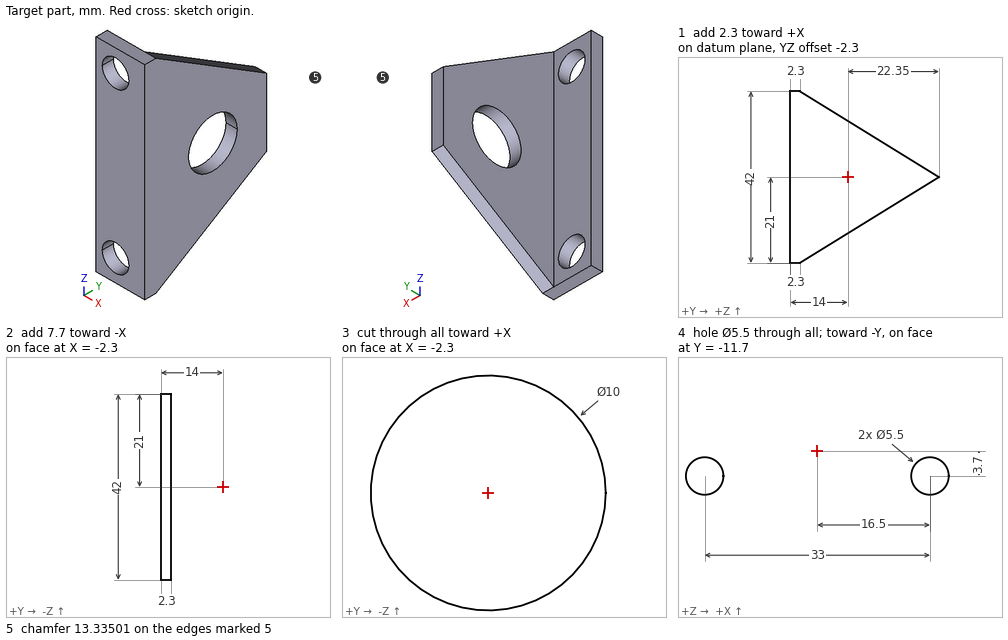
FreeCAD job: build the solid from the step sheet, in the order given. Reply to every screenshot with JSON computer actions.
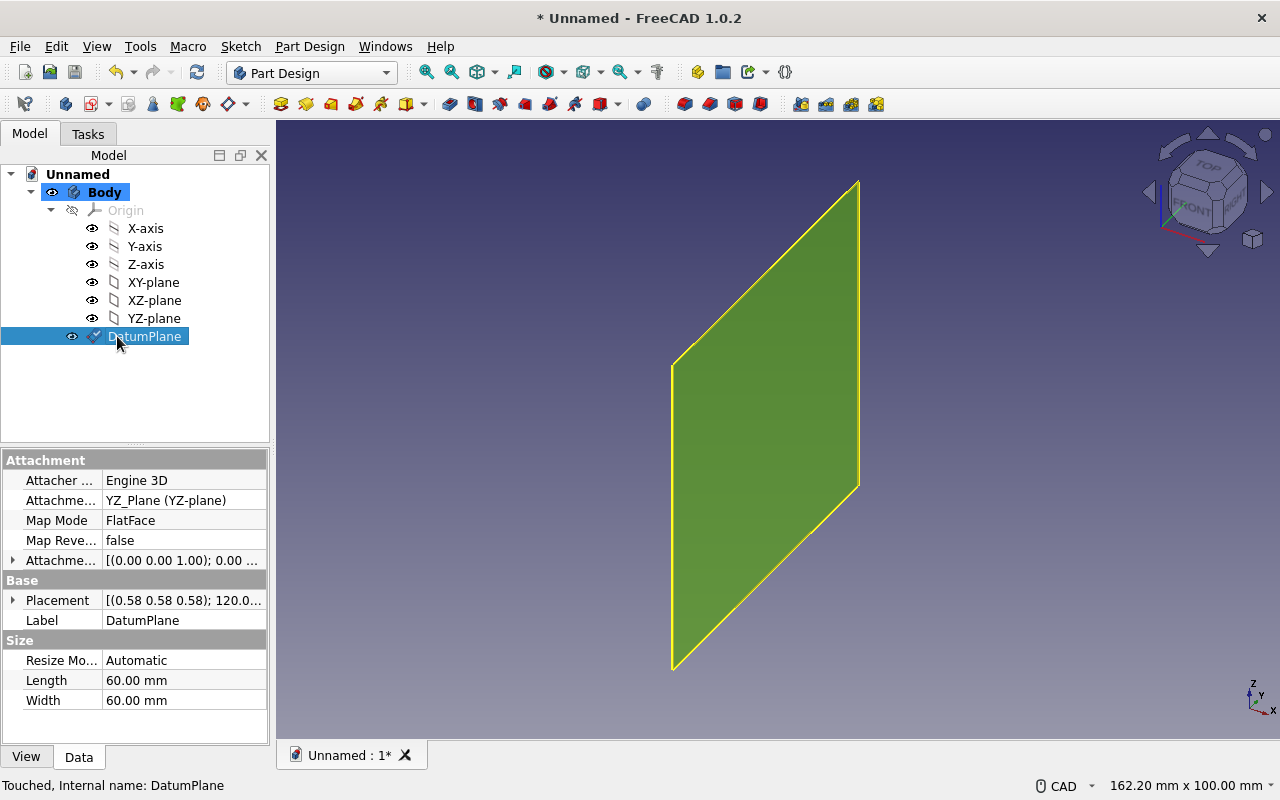
{"action": "left_click", "coordinate": [90, 104]}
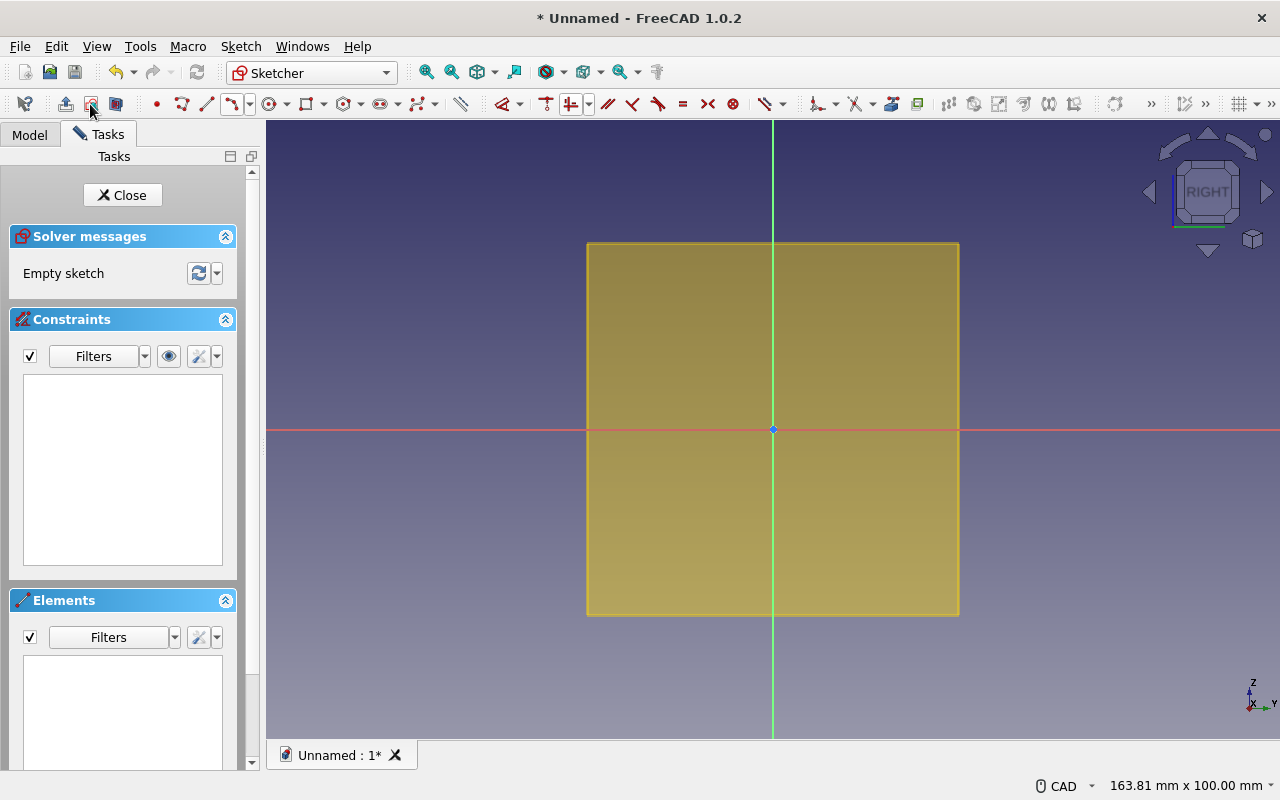
{"action": "scroll", "coordinate": [991, 429], "scroll_direction": "up", "scroll_amount": 2}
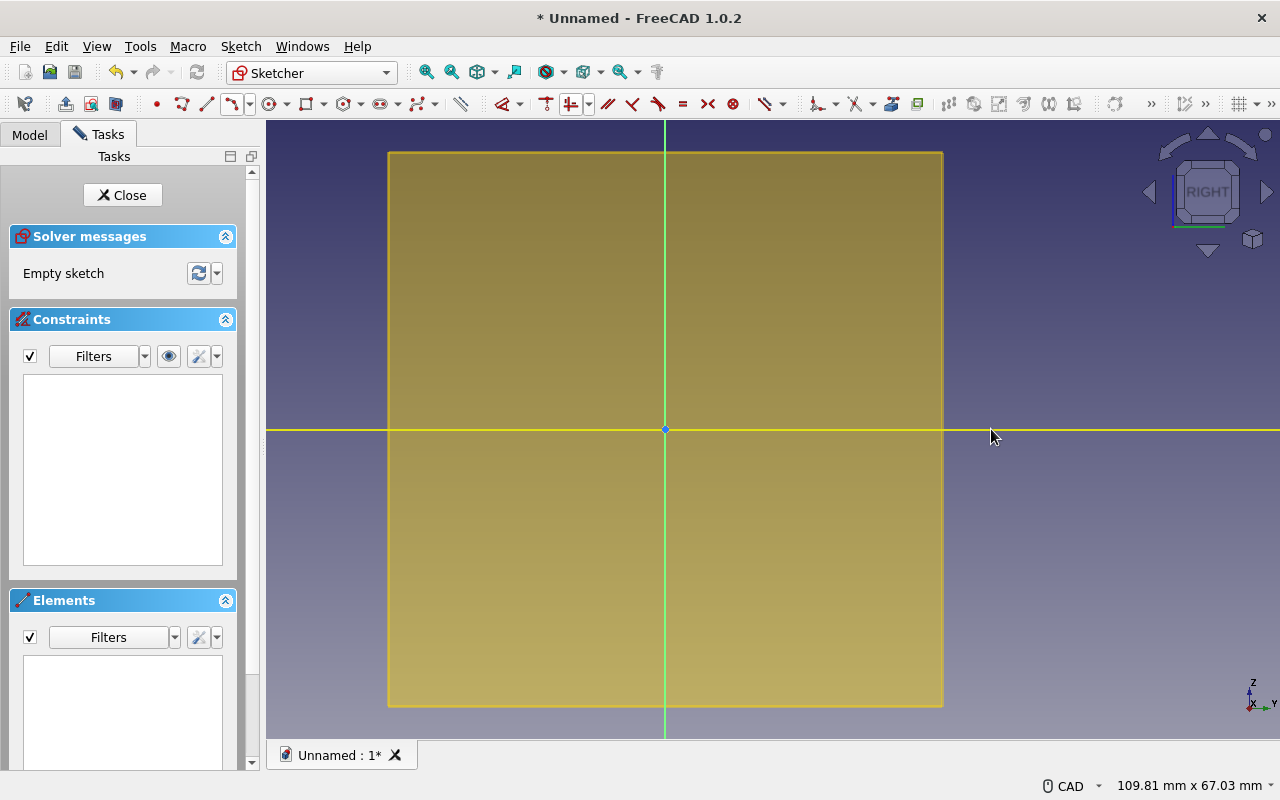
{"action": "key", "text": "g m"}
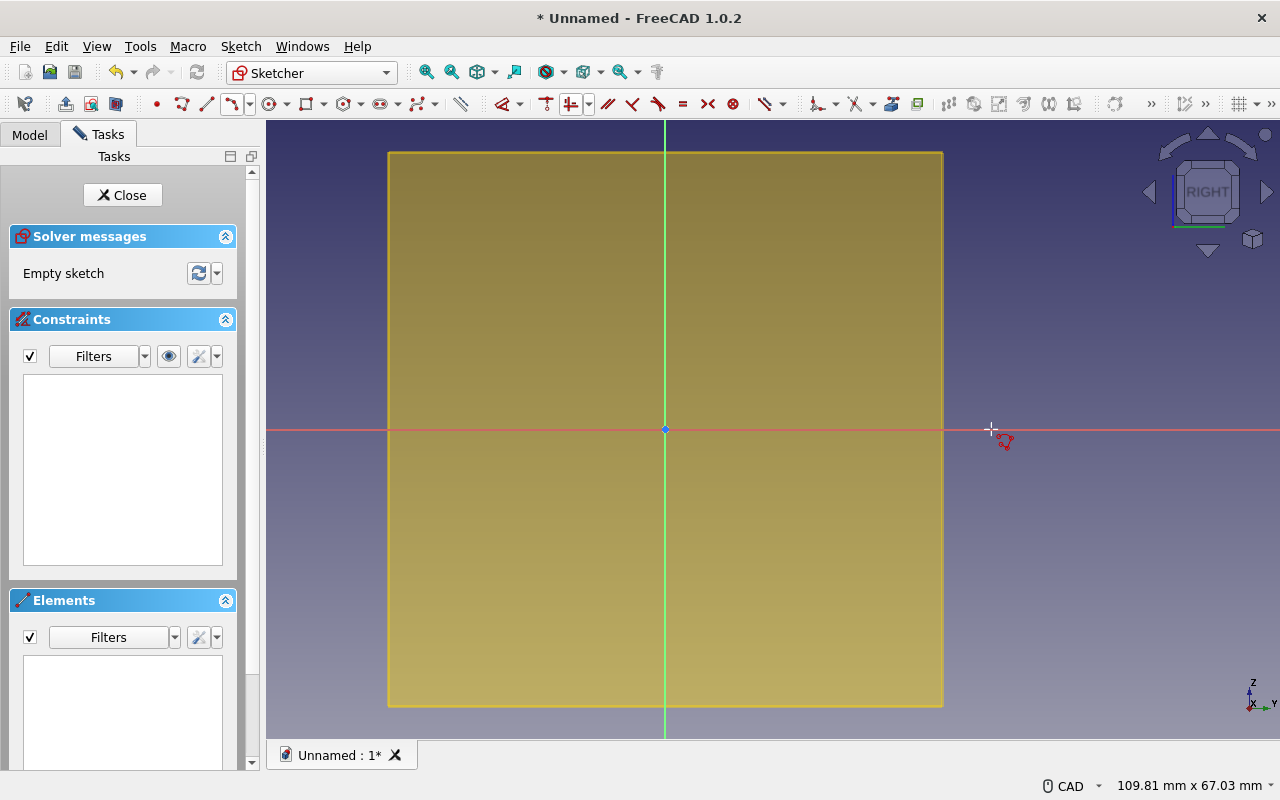
{"action": "left_click", "coordinate": [872, 430]}
{"action": "left_click", "coordinate": [557, 623]}
{"action": "left_click", "coordinate": [536, 623]}
{"action": "left_click", "coordinate": [536, 236]}
{"action": "left_click", "coordinate": [557, 236]}
{"action": "left_click", "coordinate": [872, 430]}
{"action": "key", "text": "Escape"}
{"action": "key", "text": "Escape"}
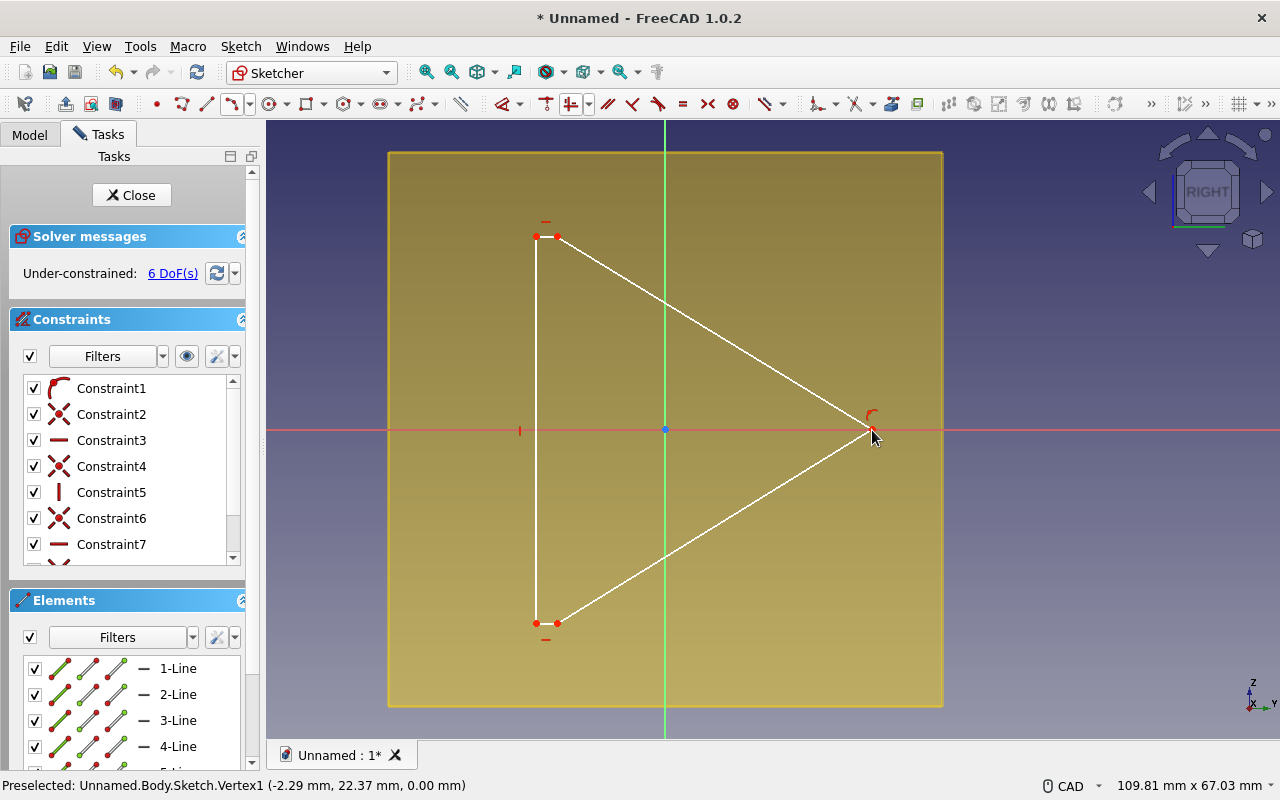
{"action": "left_click", "coordinate": [536, 508]}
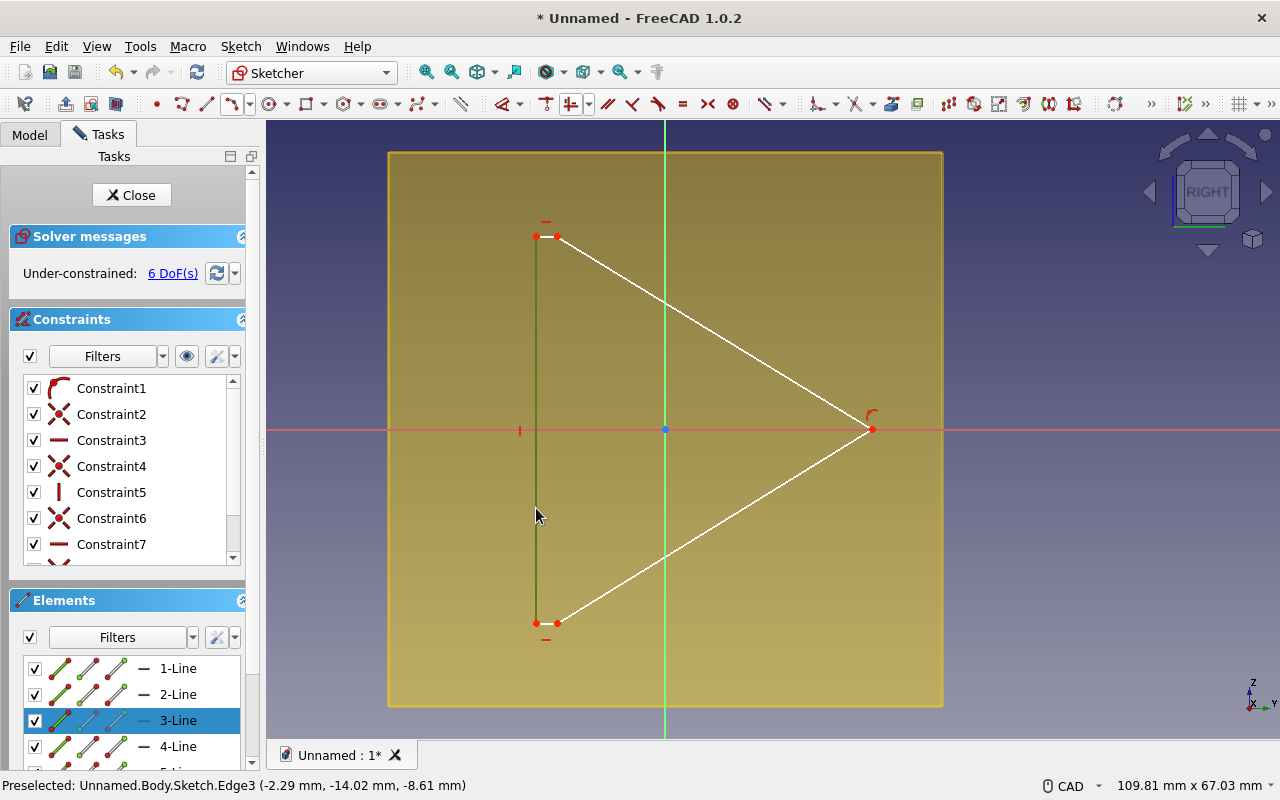
{"action": "key", "text": "i"}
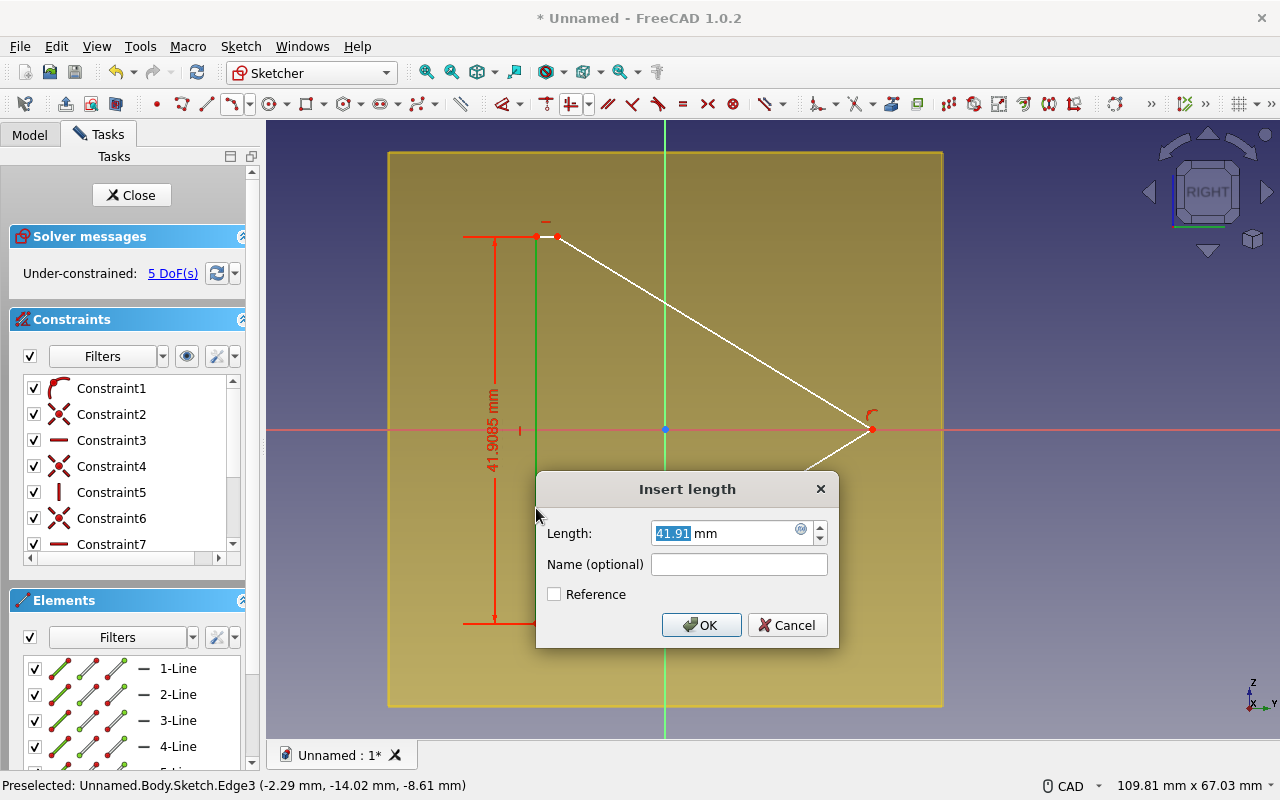
{"action": "type", "text": "42"}
{"action": "key", "text": "Return"}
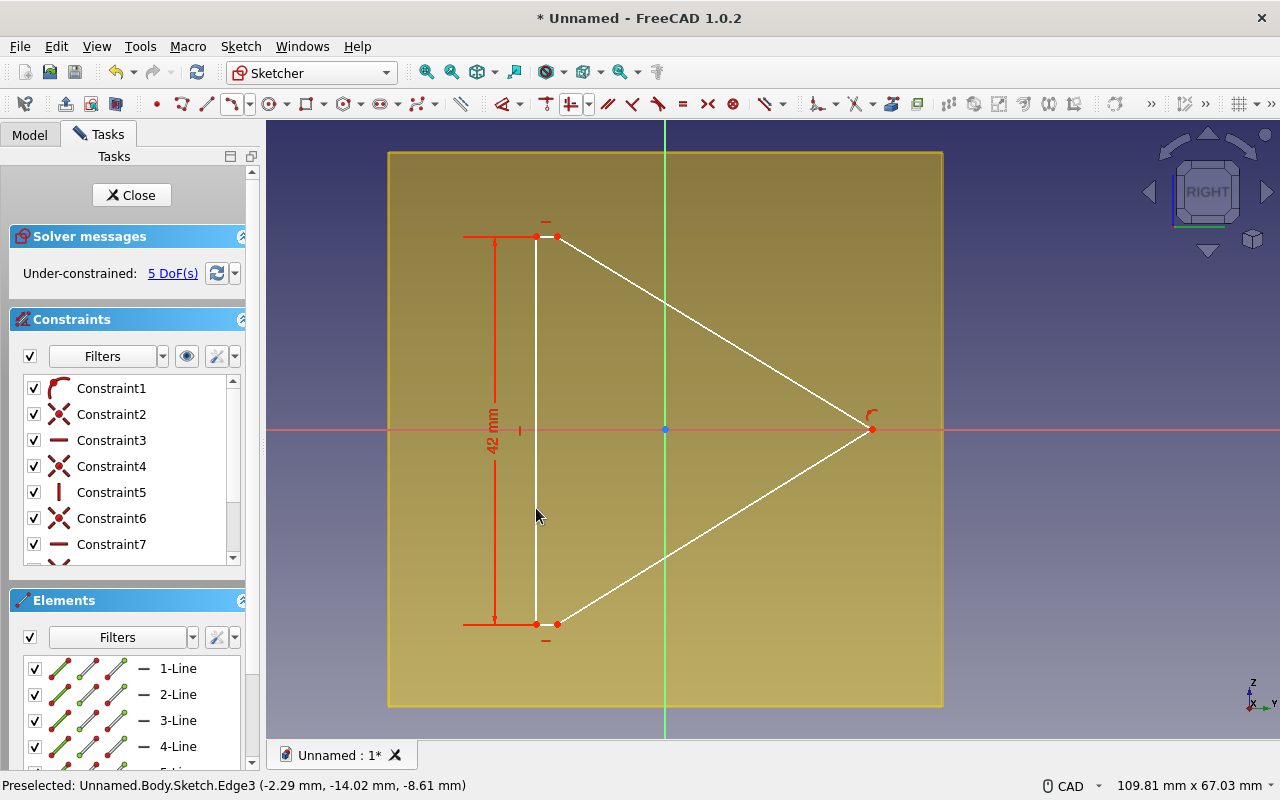
{"action": "scroll", "coordinate": [546, 625], "scroll_direction": "up", "scroll_amount": 4}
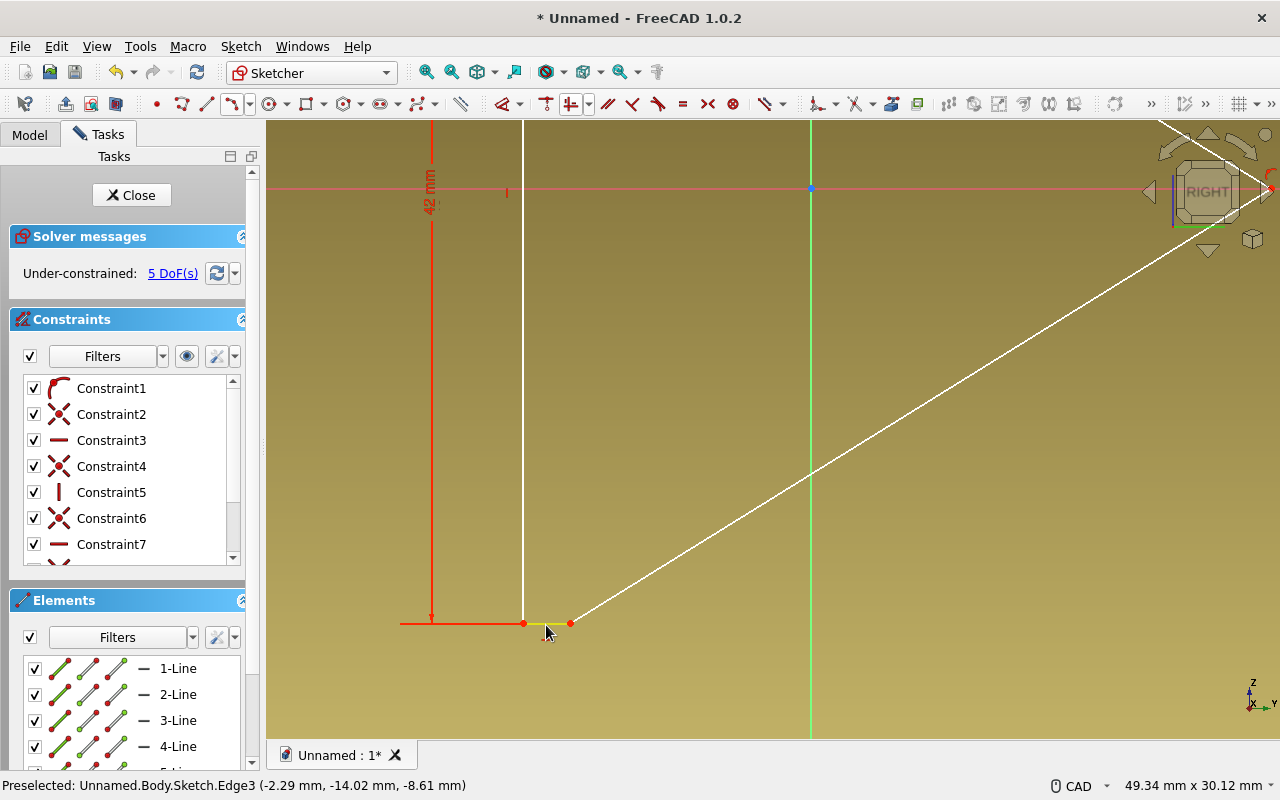
{"action": "left_click", "coordinate": [547, 624]}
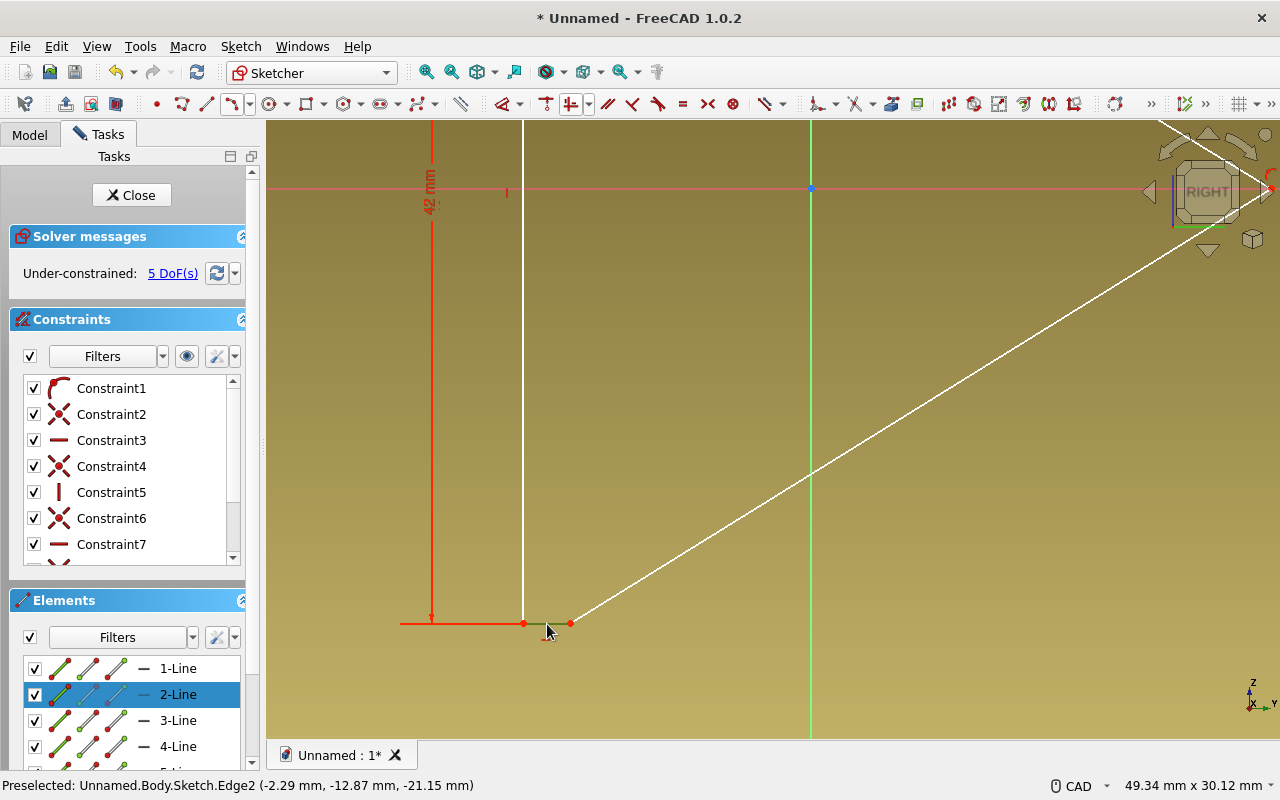
{"action": "key", "text": "l"}